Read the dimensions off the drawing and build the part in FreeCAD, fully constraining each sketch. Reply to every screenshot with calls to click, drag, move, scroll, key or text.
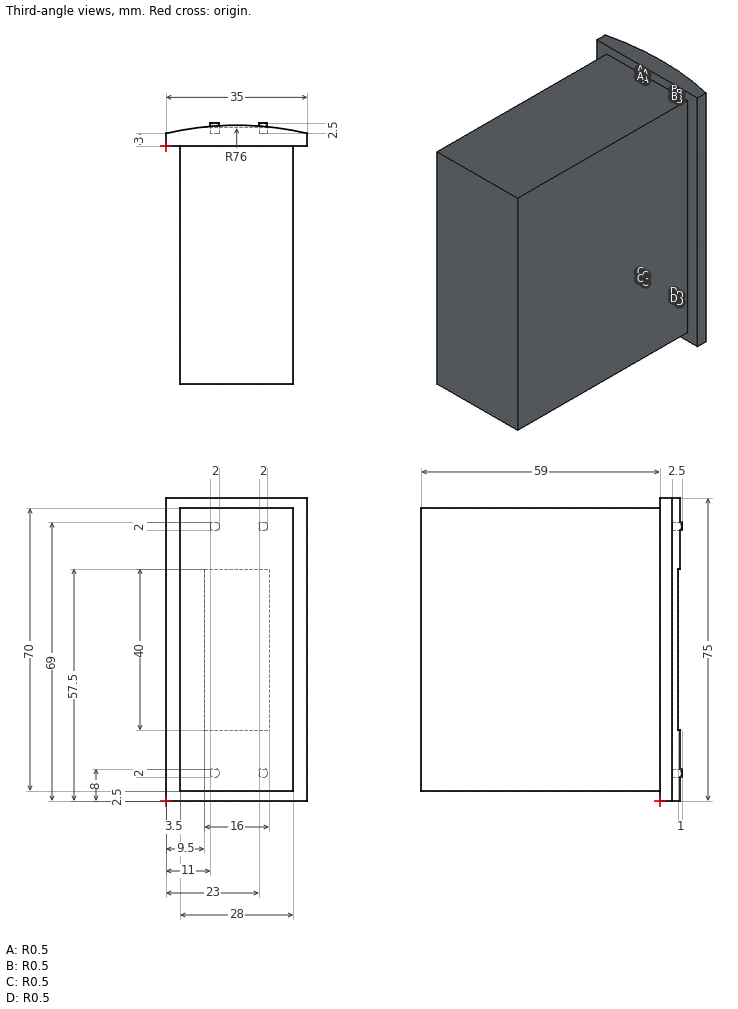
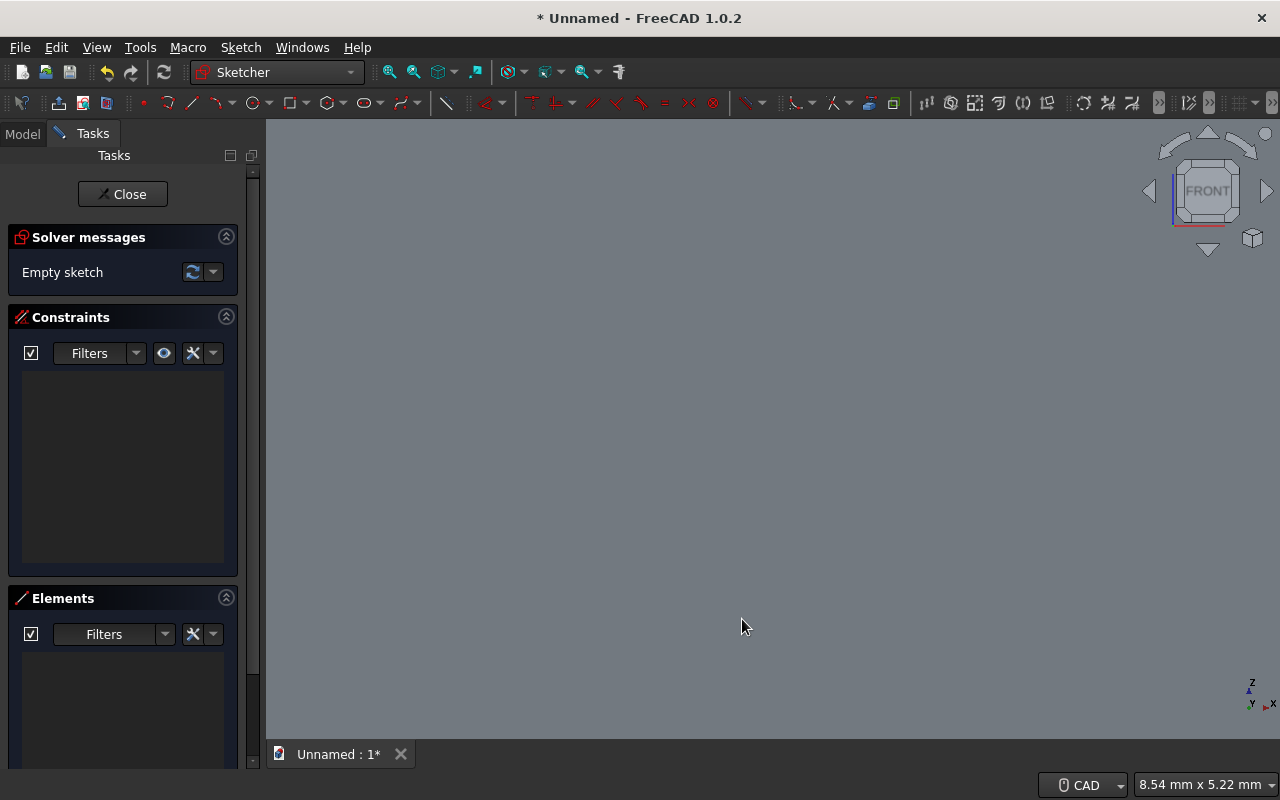
scroll(701, 380, up, 3)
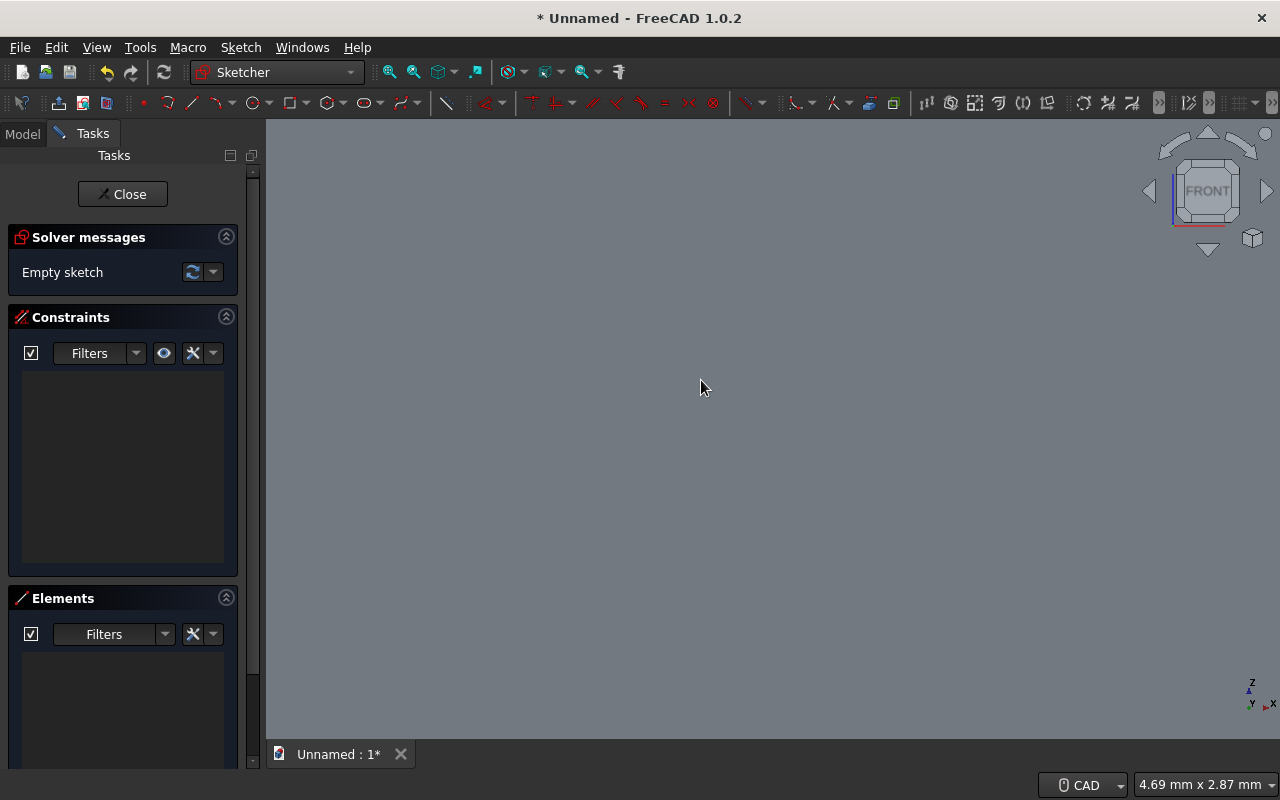
click(290, 104)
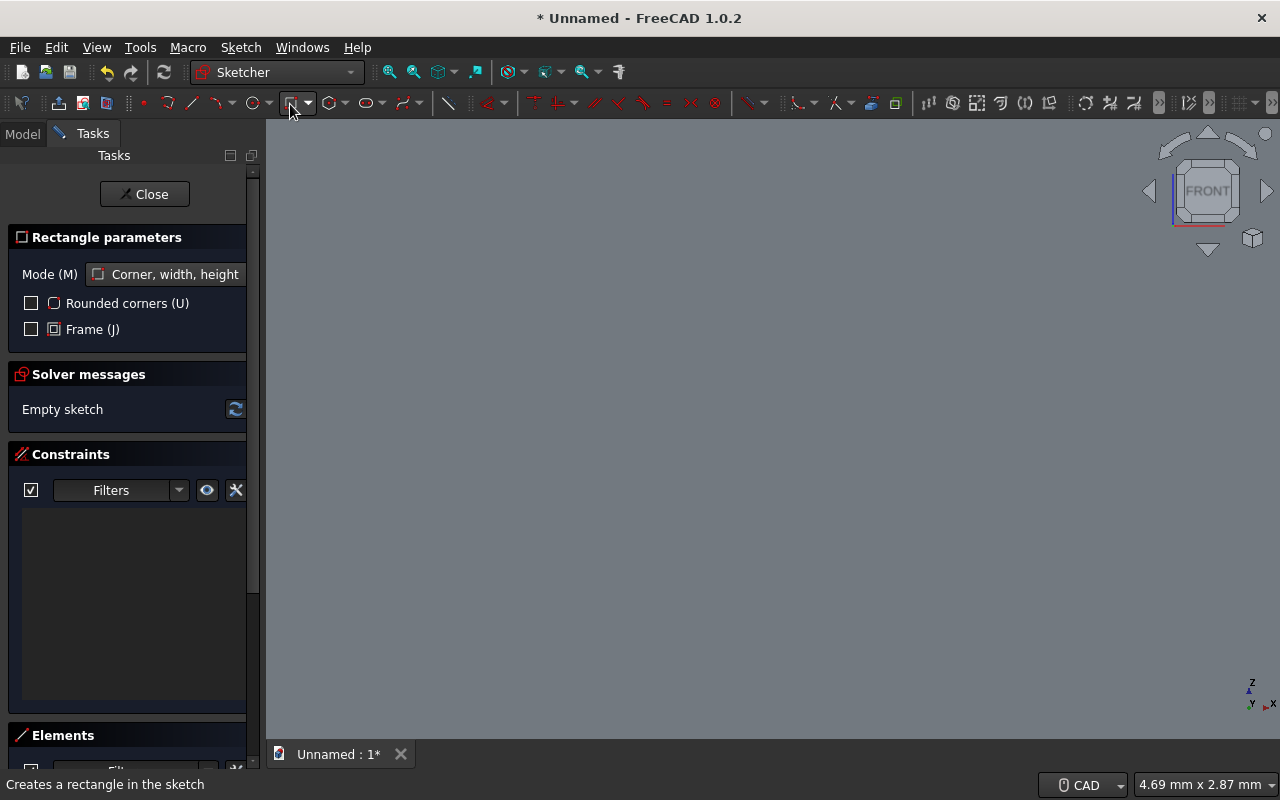
click(488, 213)
click(920, 645)
key(Escape)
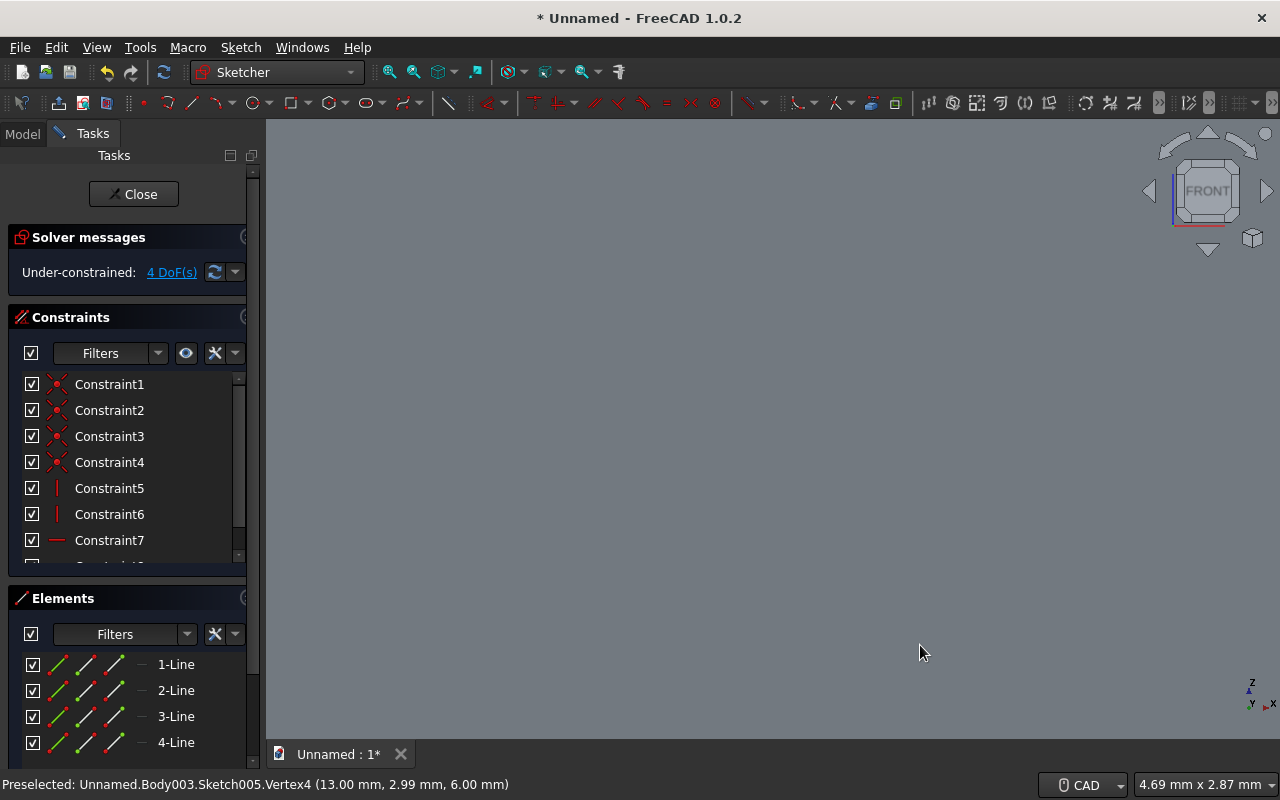
key(d)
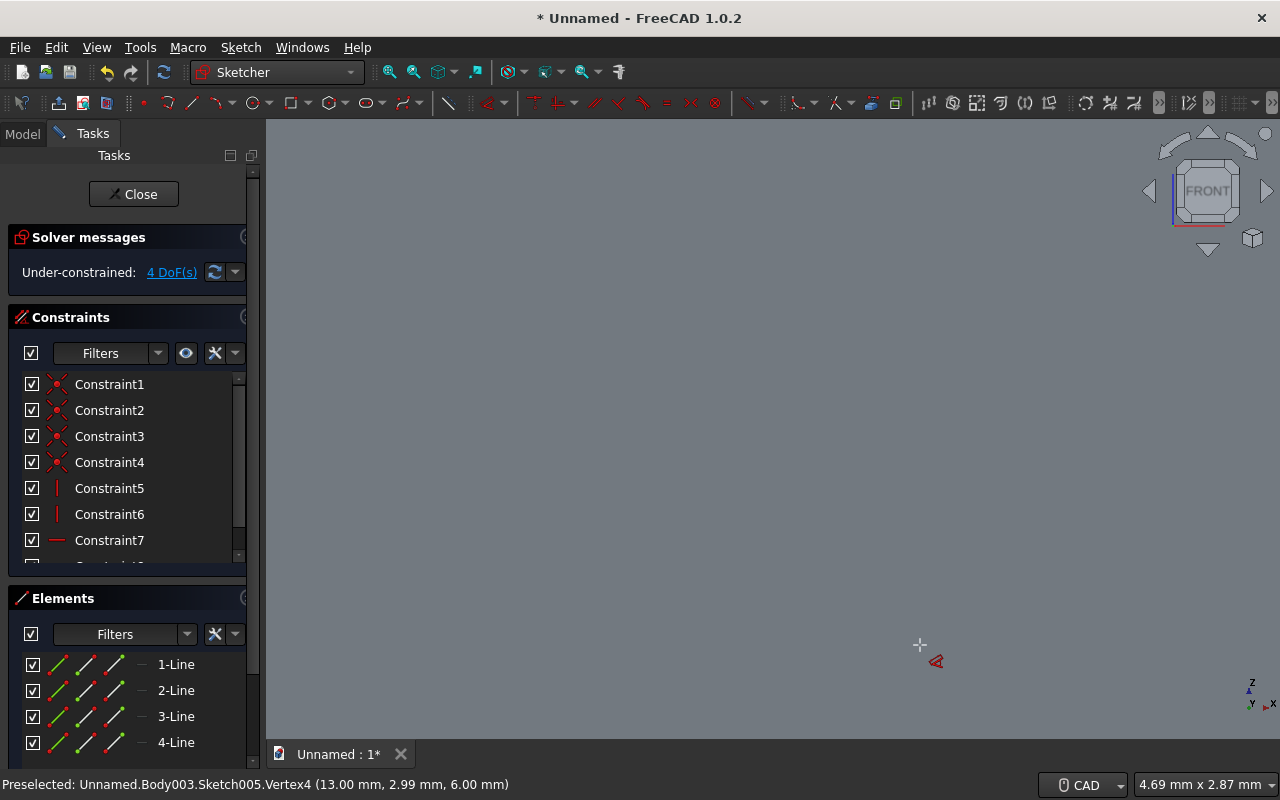
click(488, 344)
click(454, 430)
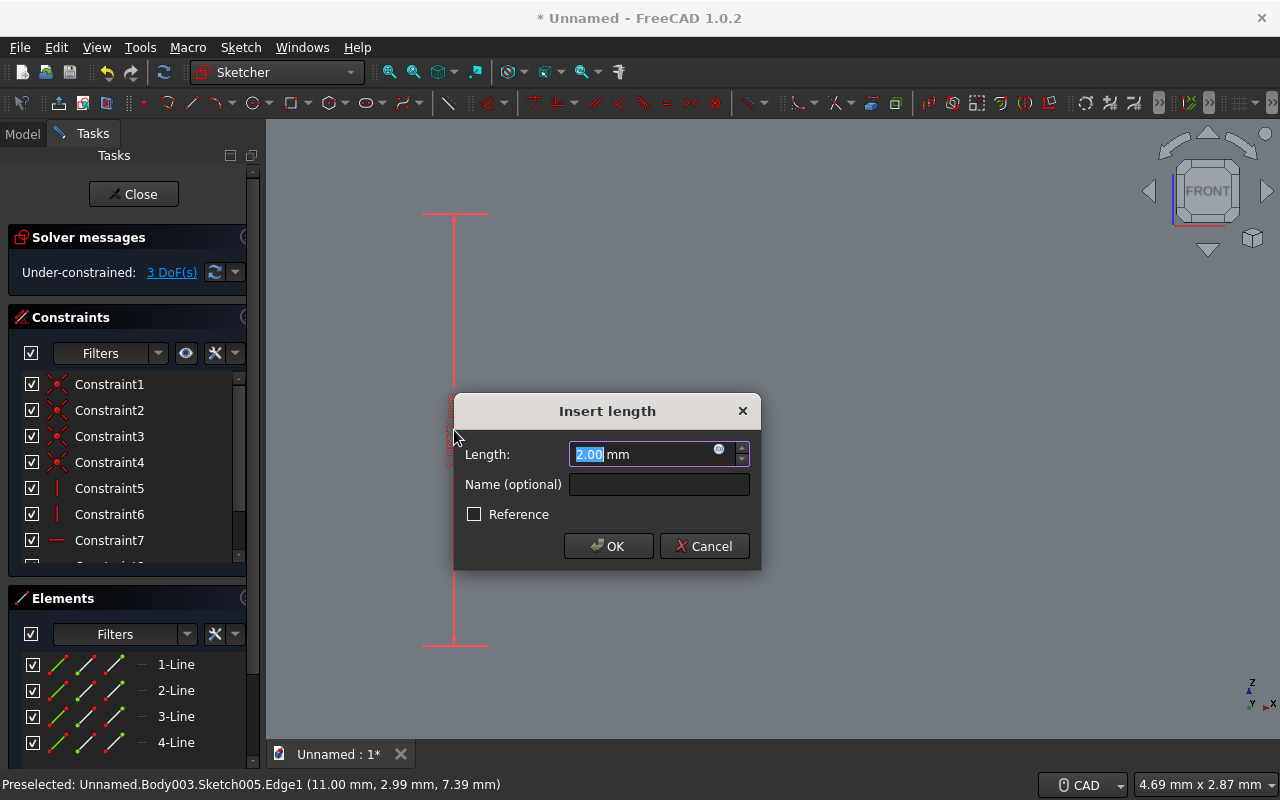
text(2)
key(Return)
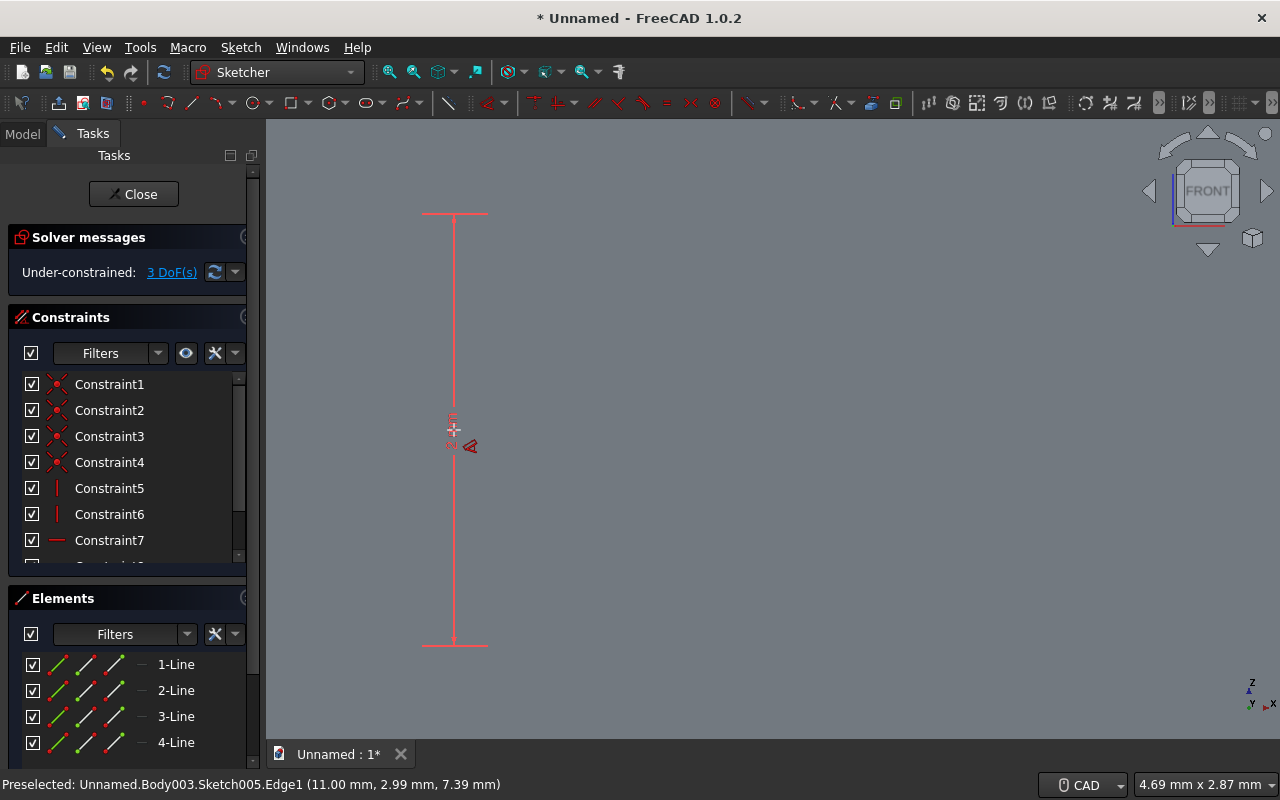
click(618, 646)
click(704, 680)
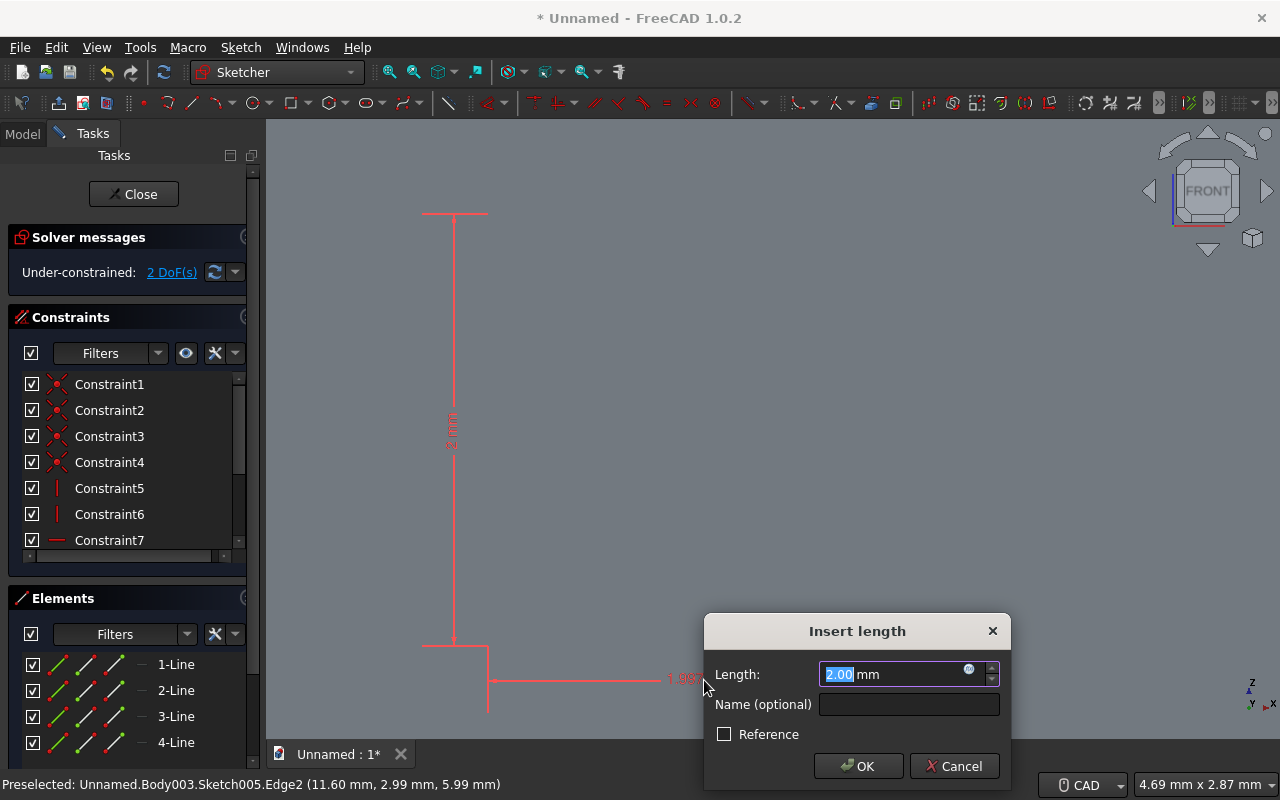
text(2)
key(Return)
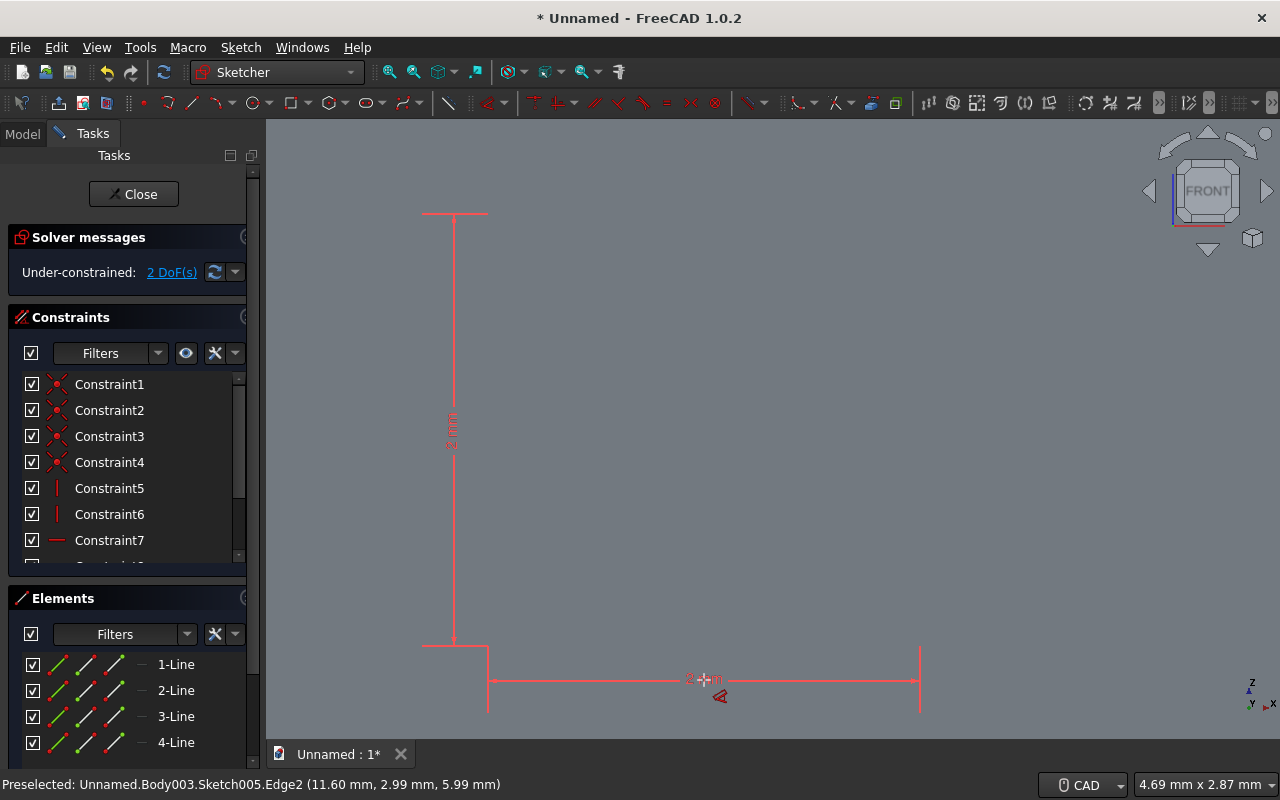
click(488, 214)
click(522, 463)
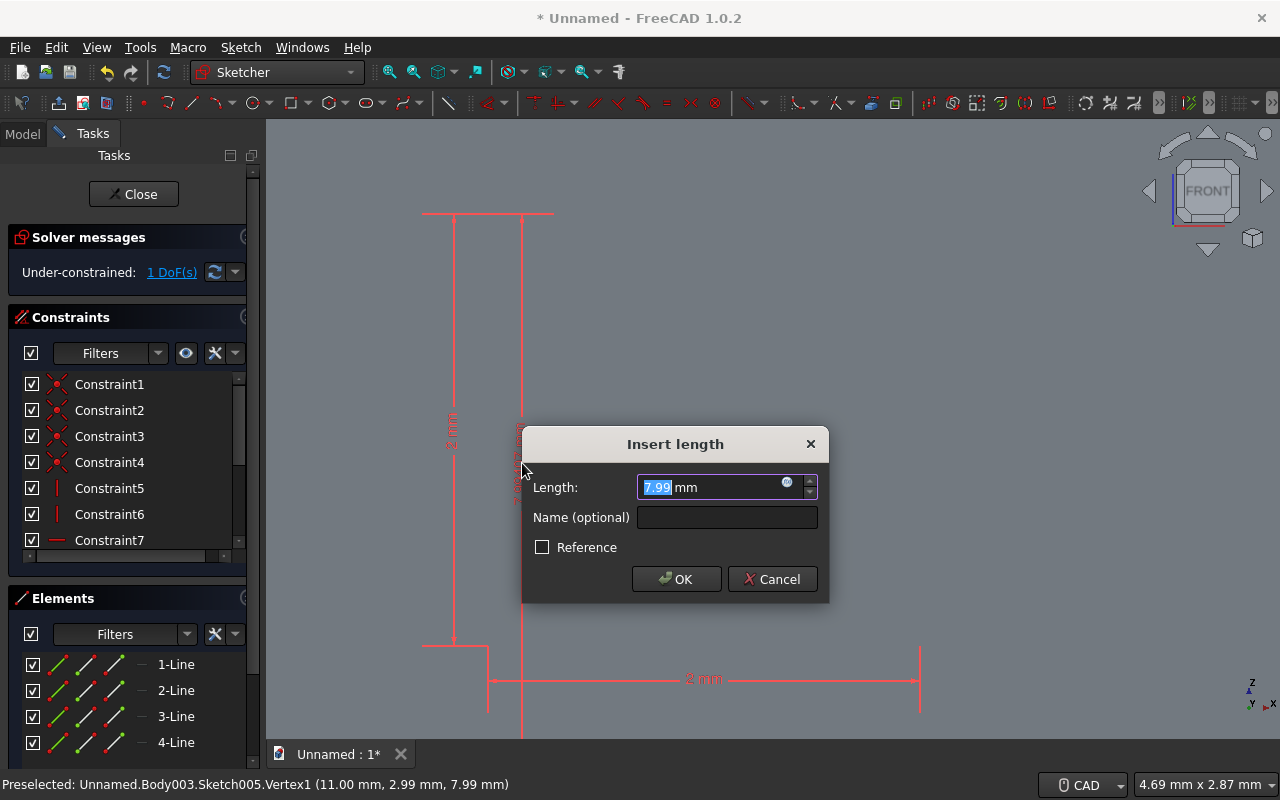
text(8)
key(Return)